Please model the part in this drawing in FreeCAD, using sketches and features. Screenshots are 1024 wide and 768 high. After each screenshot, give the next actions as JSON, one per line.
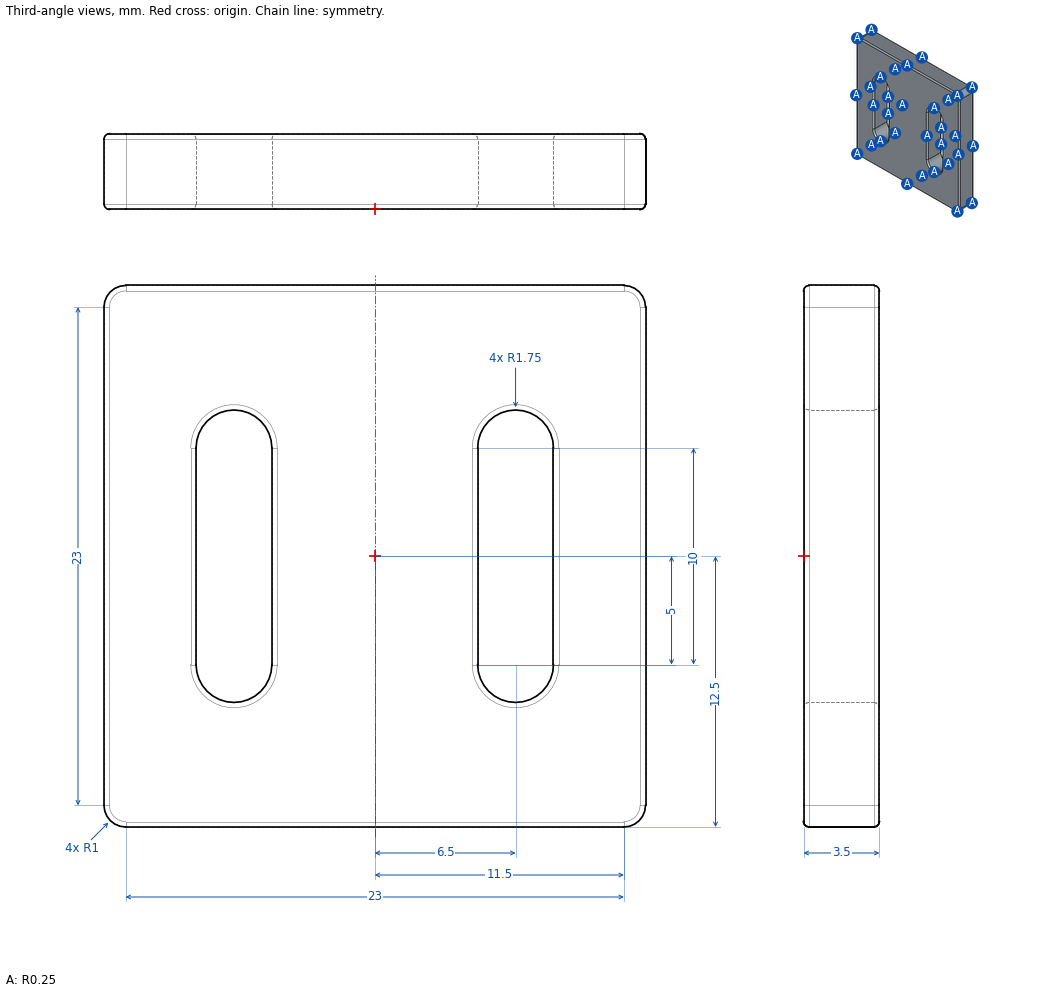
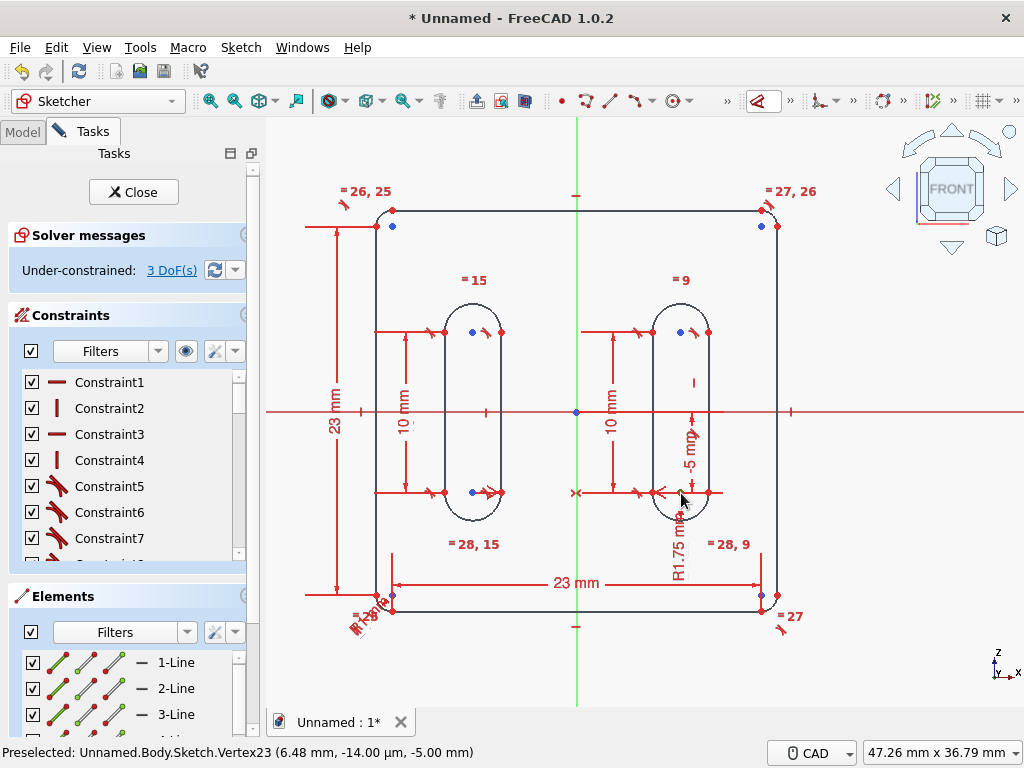
{"action": "key", "text": "l"}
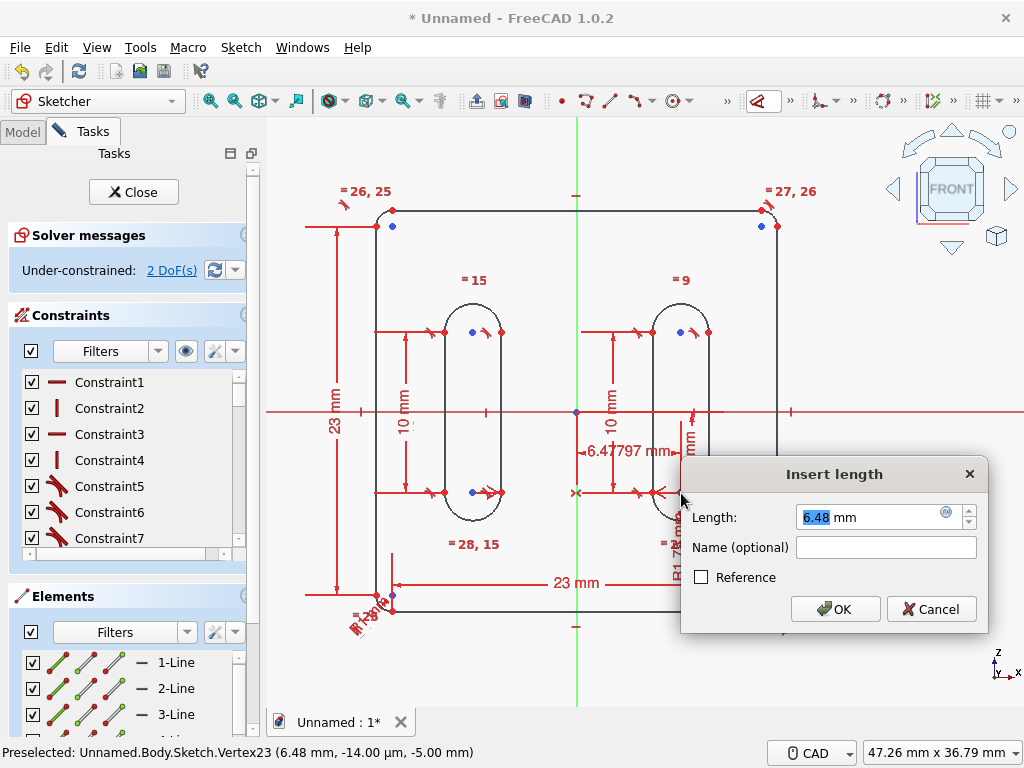
{"action": "type", "text": "6.5"}
{"action": "key", "text": "Return"}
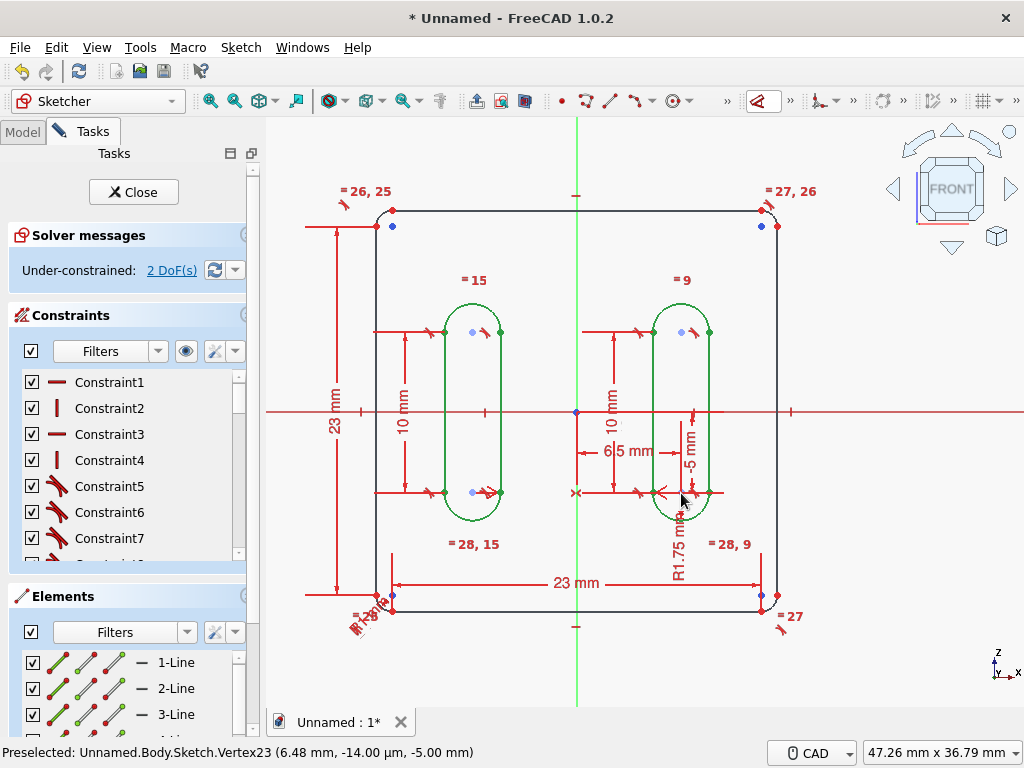
{"action": "left_click", "coordinate": [761, 612]}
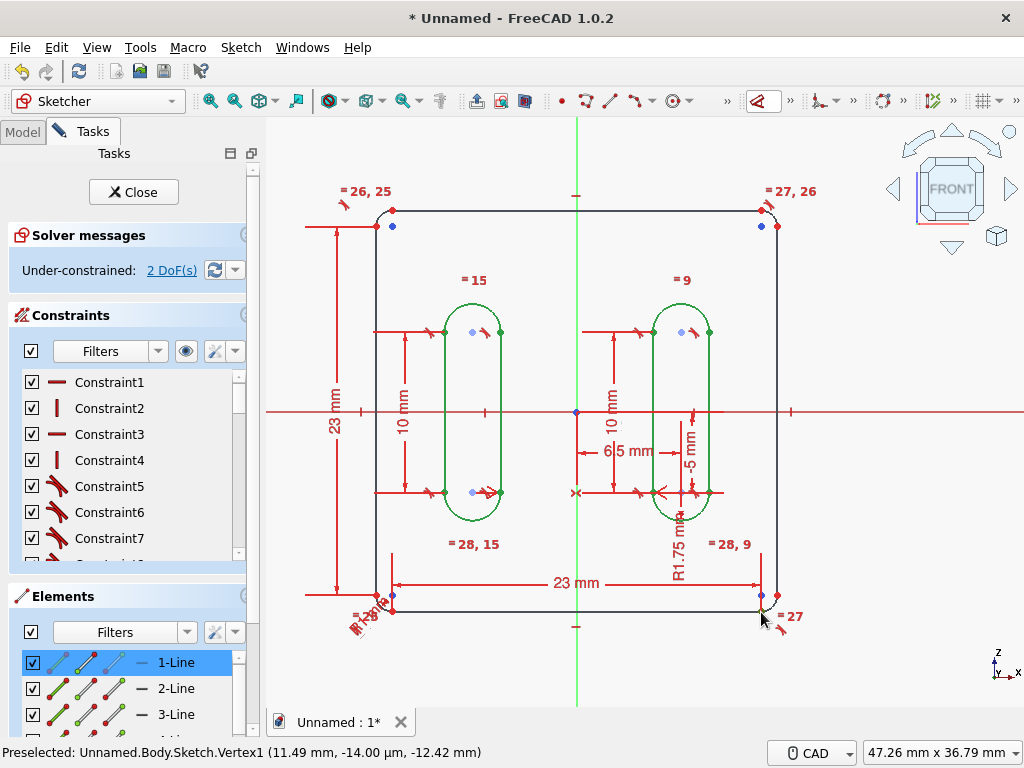
{"action": "key", "text": "l"}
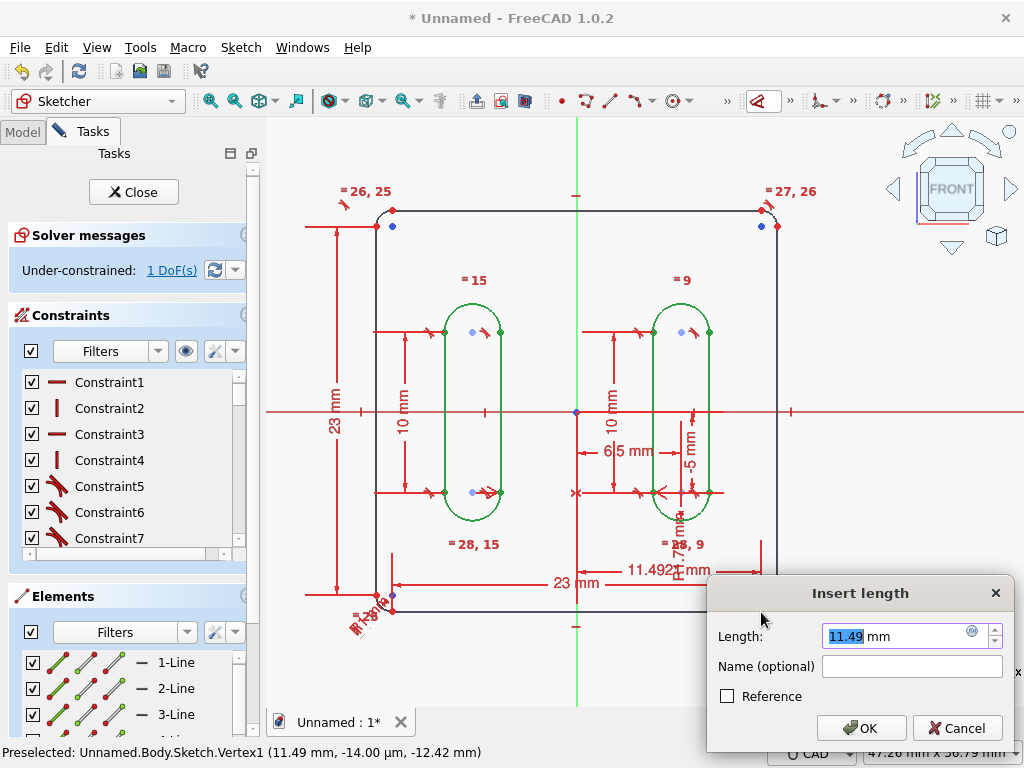
{"action": "type", "text": "11.5"}
{"action": "key", "text": "Return"}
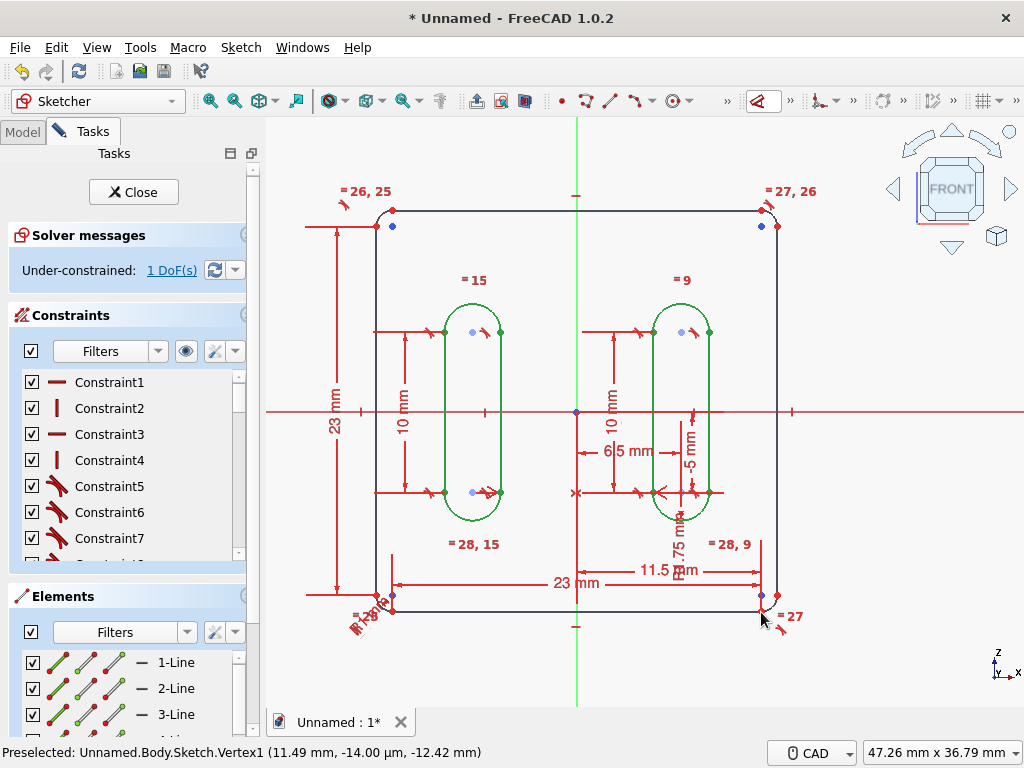
{"action": "left_click", "coordinate": [761, 612]}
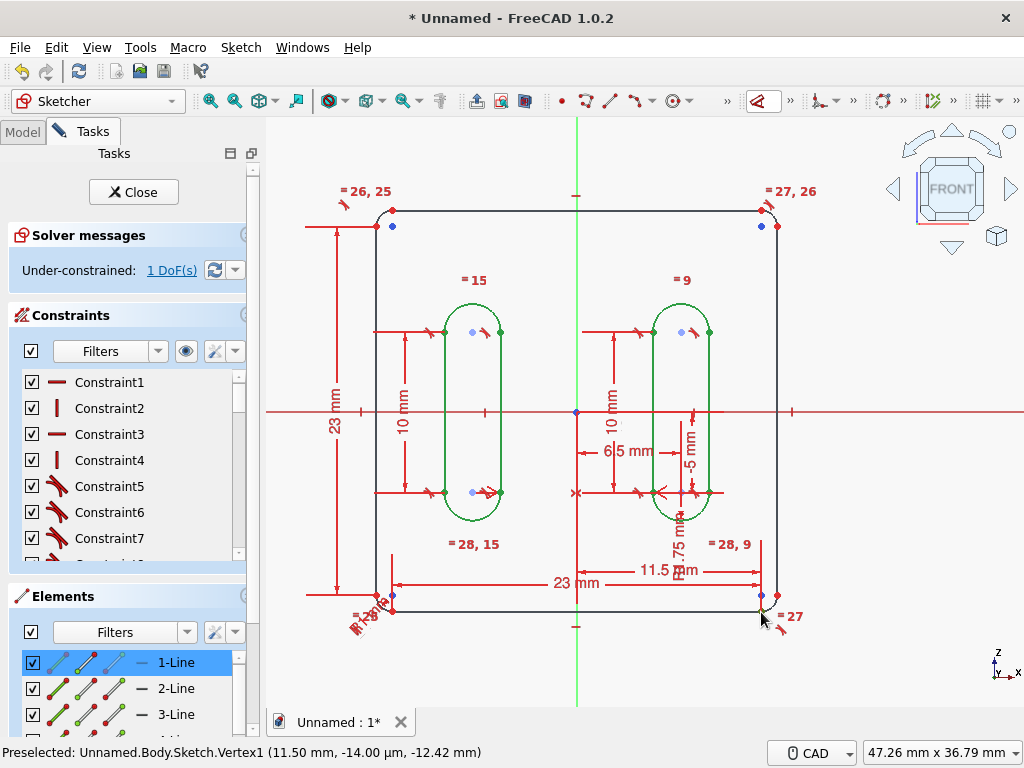
{"action": "key", "text": "i"}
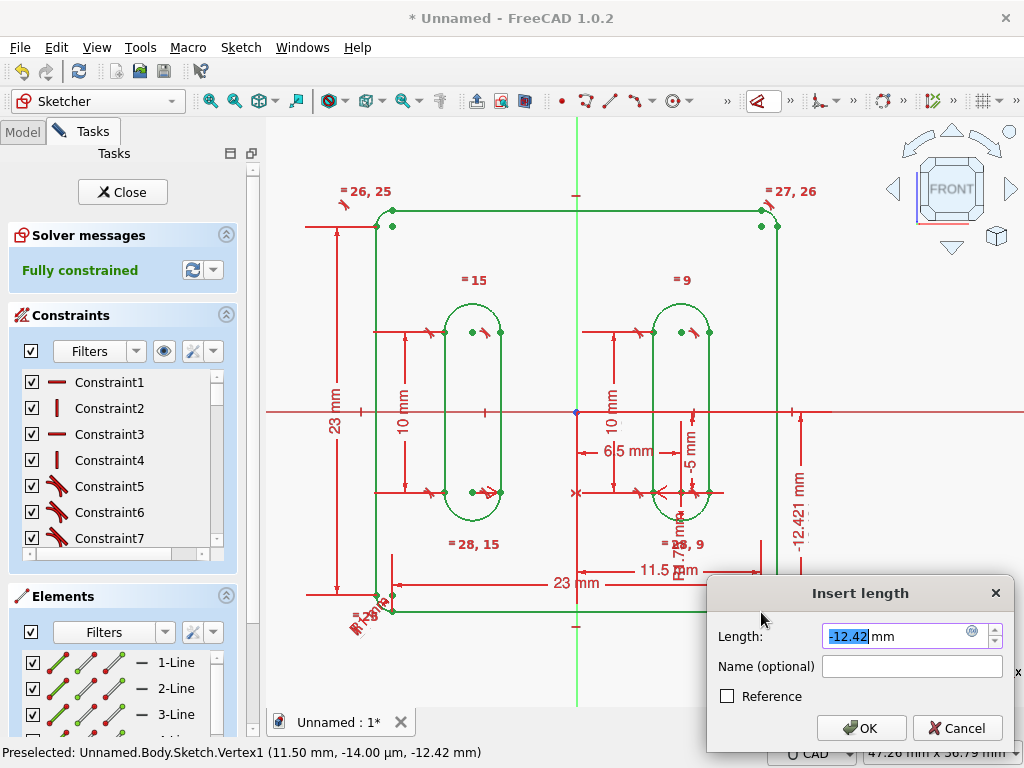
{"action": "type", "text": "-12.5"}
{"action": "key", "text": "Return"}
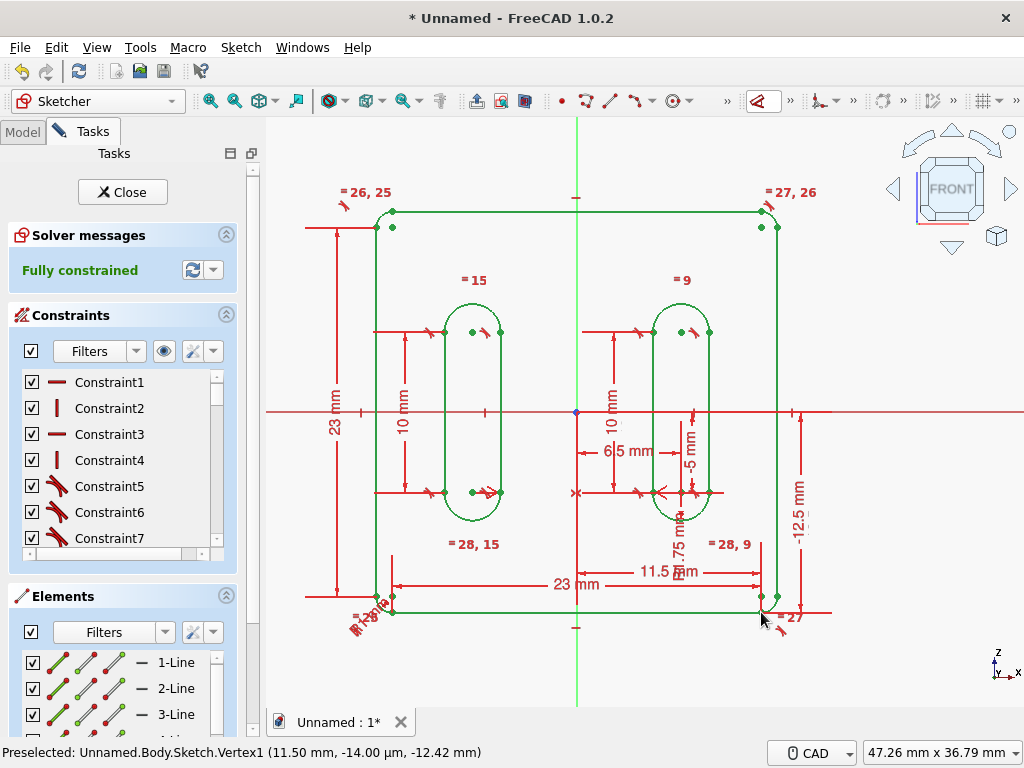
{"action": "left_click", "coordinate": [123, 192]}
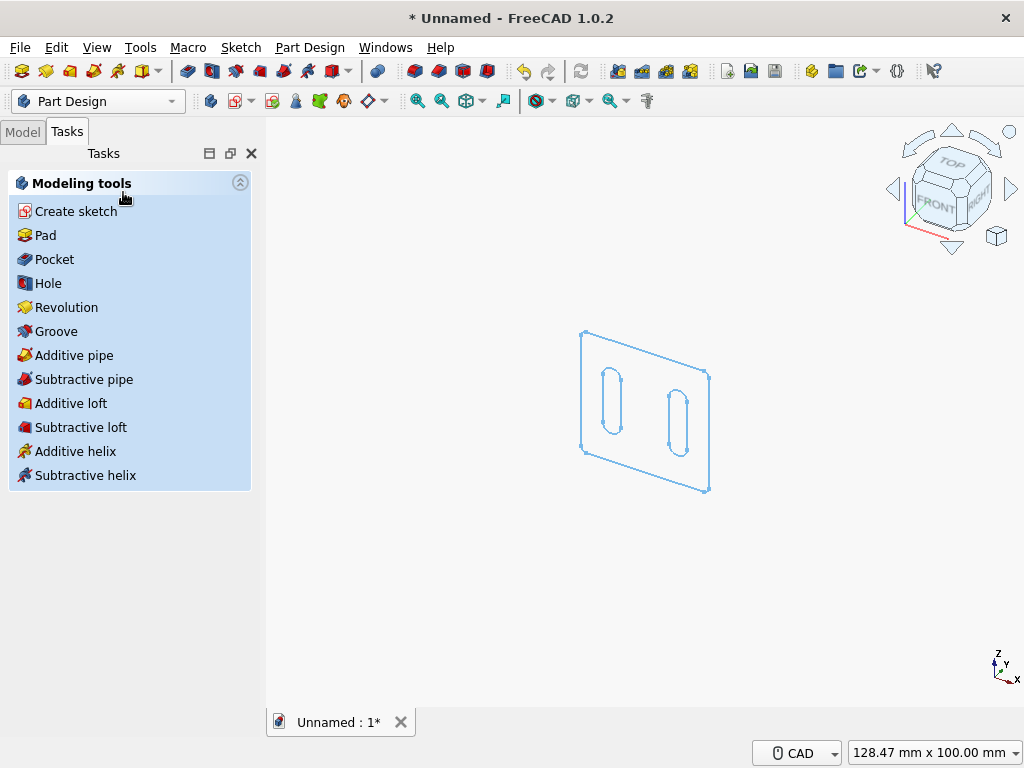
{"action": "left_click", "coordinate": [22, 72]}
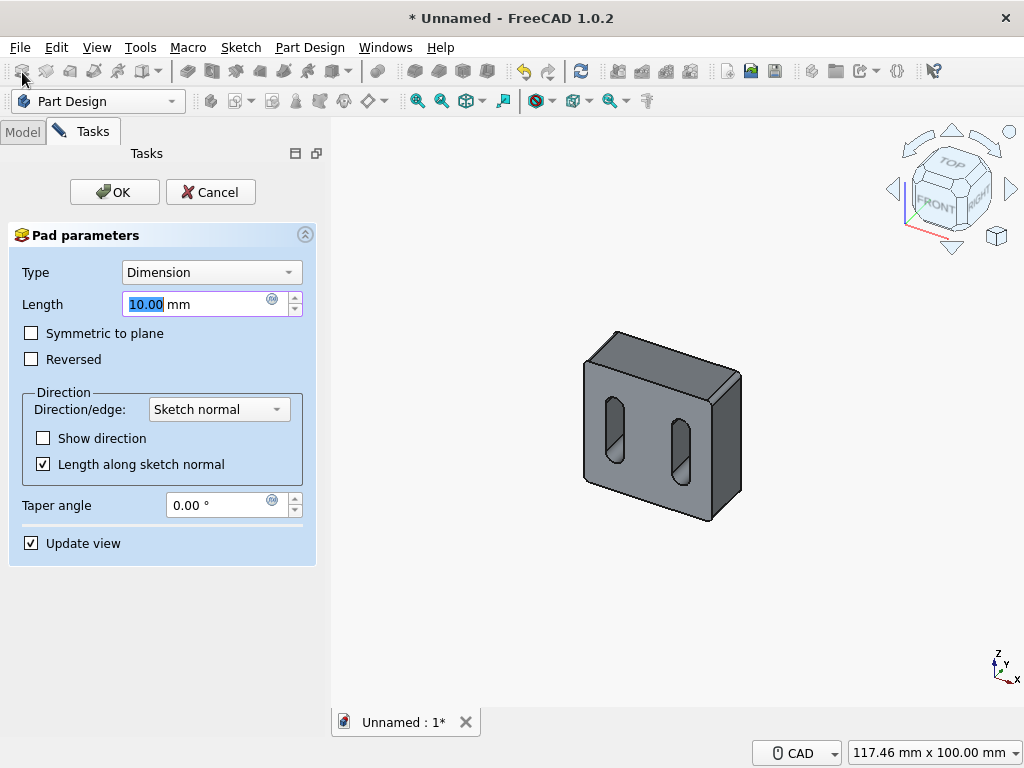
{"action": "type", "text": "3.5"}
{"action": "key", "text": "Tab"}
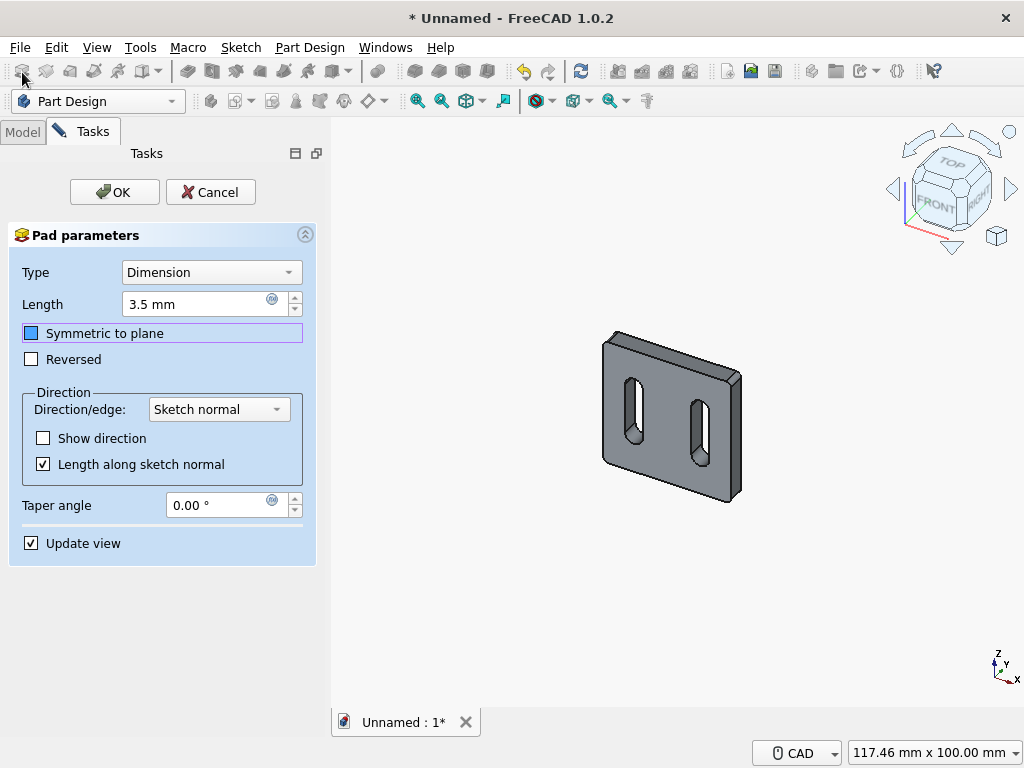
{"action": "left_click", "coordinate": [30, 359]}